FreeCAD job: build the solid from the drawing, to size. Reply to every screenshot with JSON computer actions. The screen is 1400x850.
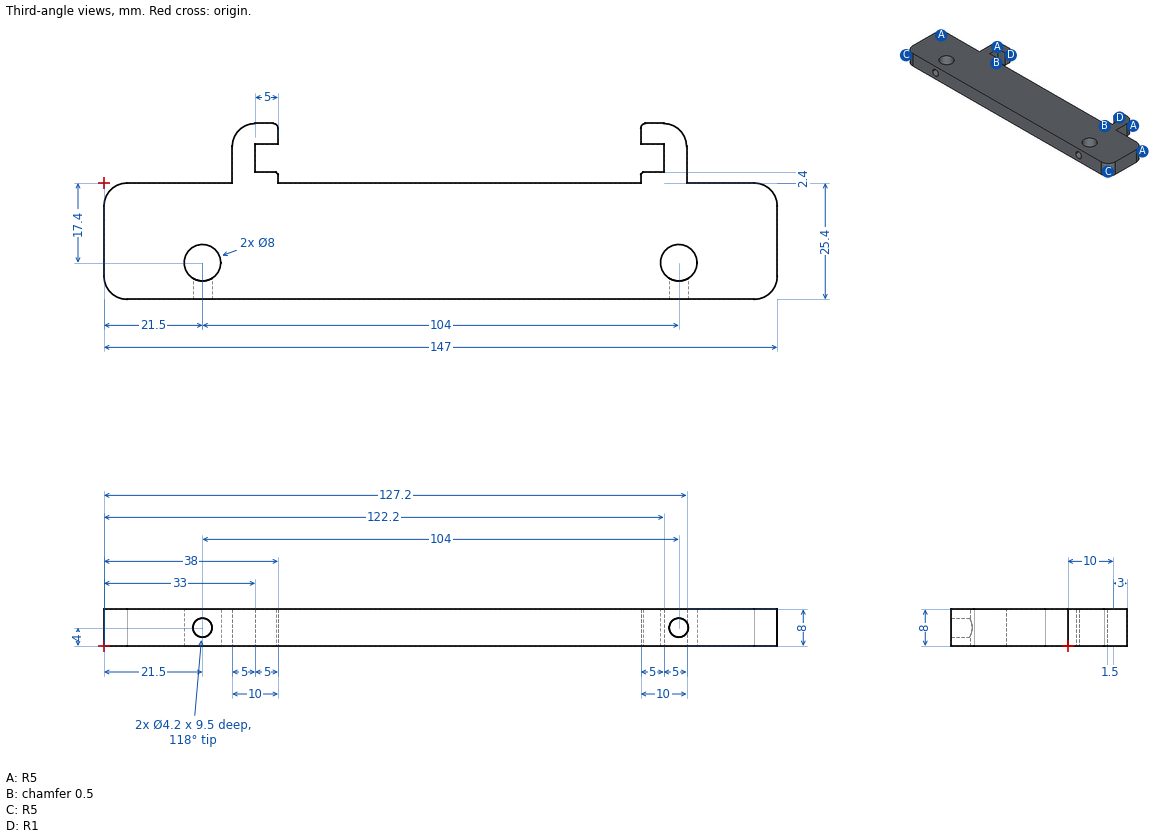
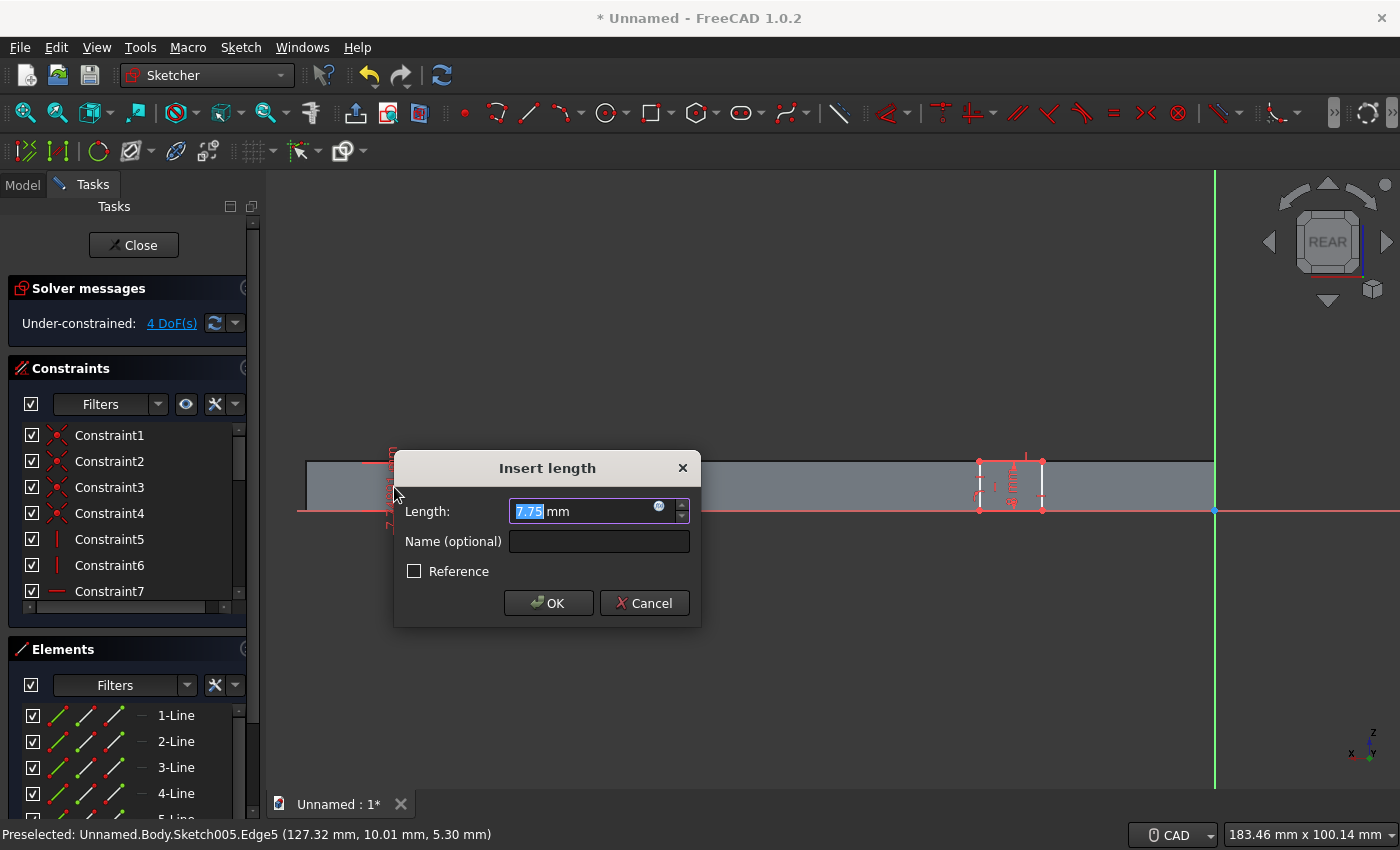
{"action": "type", "text": "8"}
{"action": "key", "text": "Return"}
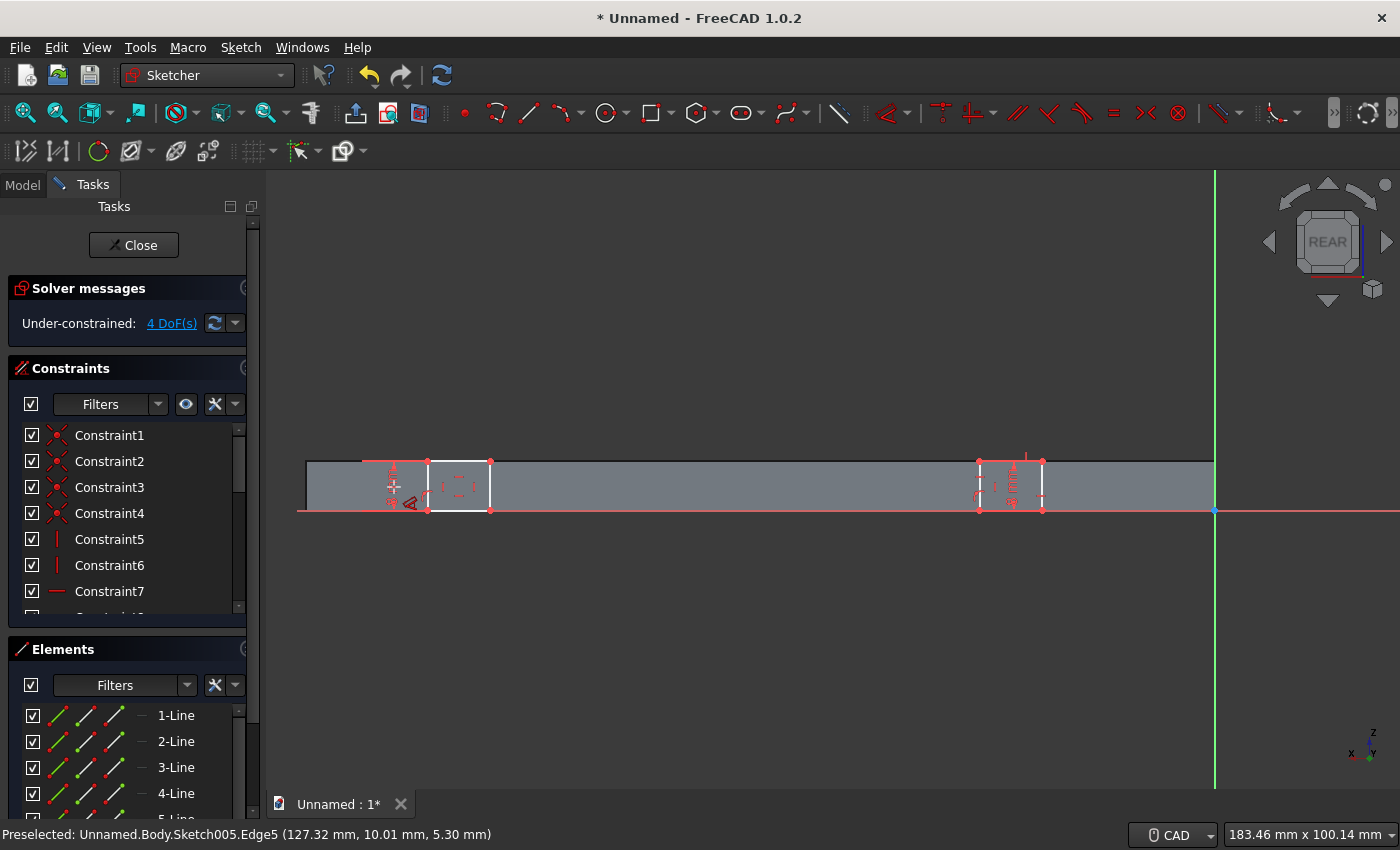
{"action": "left_click", "coordinate": [998, 511]}
{"action": "left_click", "coordinate": [1011, 545]}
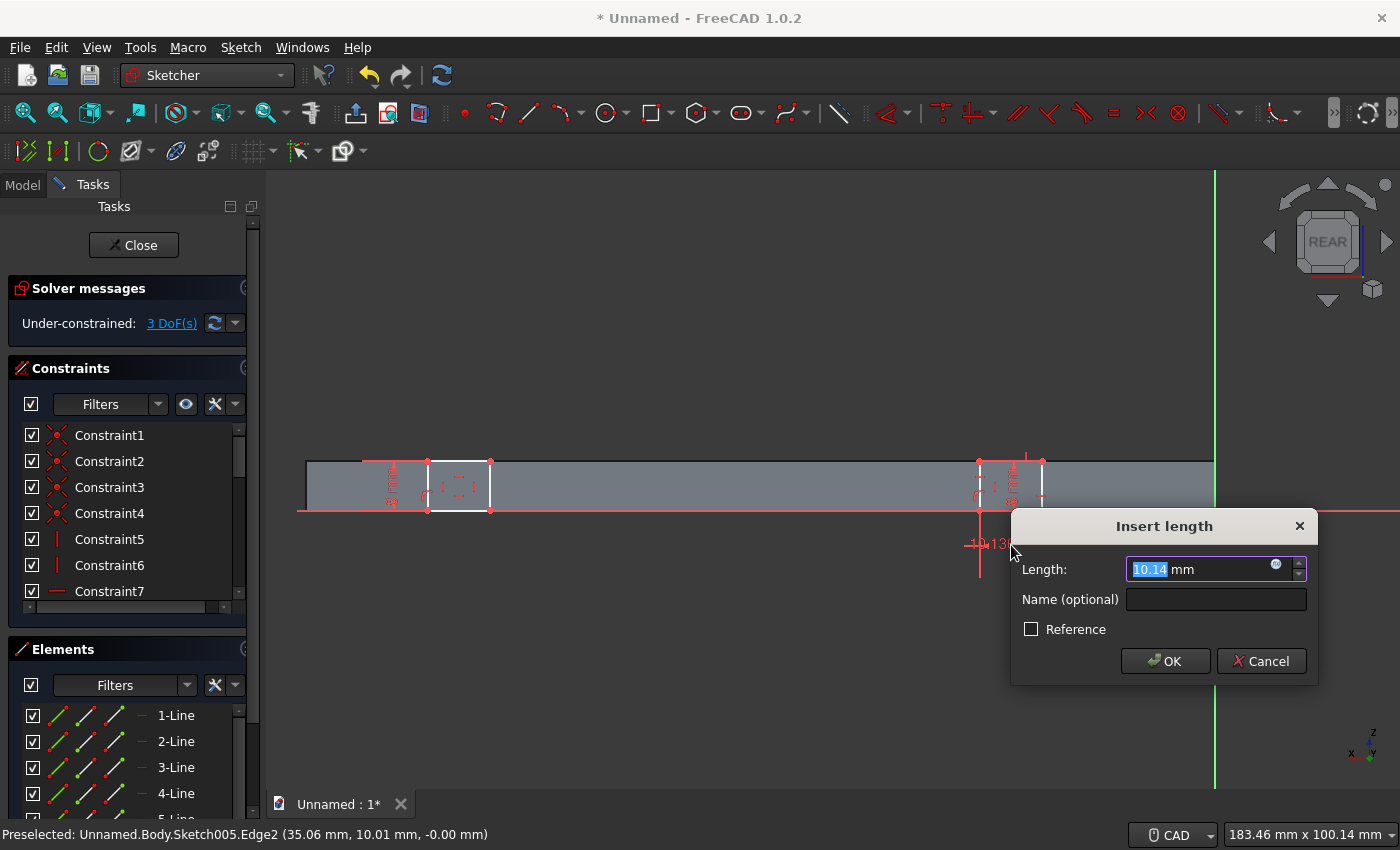
{"action": "type", "text": "10"}
{"action": "key", "text": "Return"}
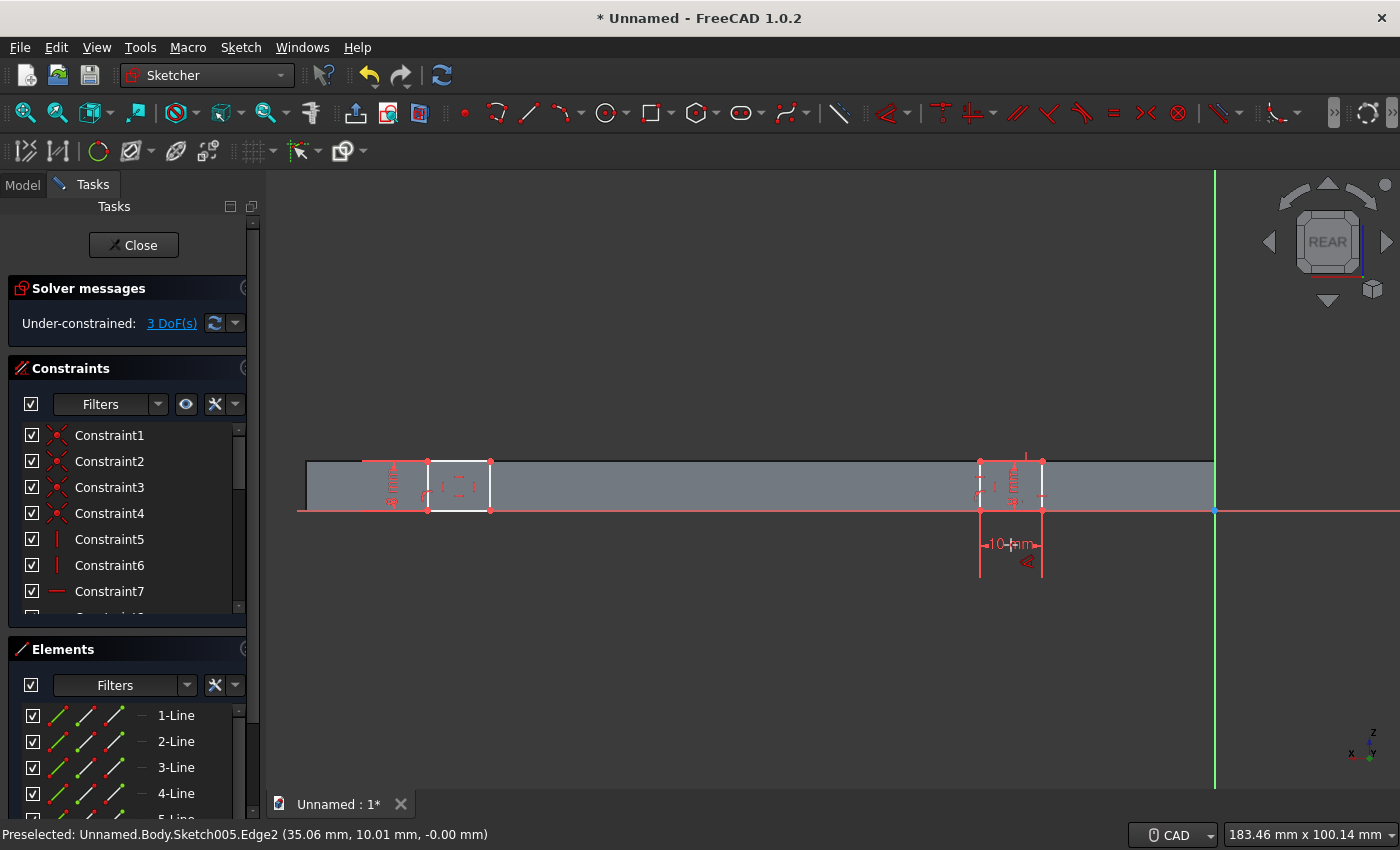
{"action": "left_click", "coordinate": [447, 511]}
{"action": "left_click", "coordinate": [459, 545]}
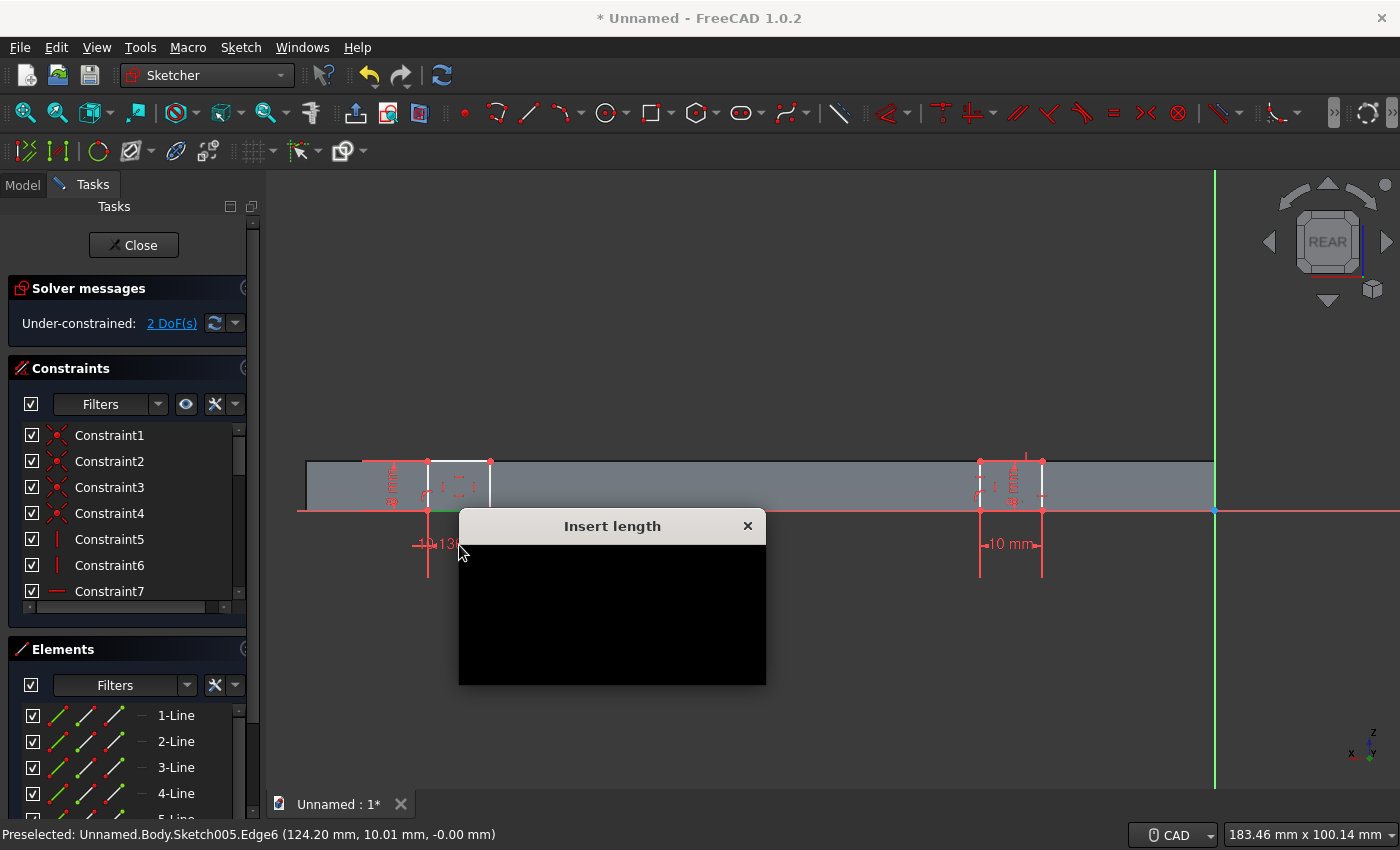
{"action": "type", "text": "10"}
{"action": "key", "text": "Return"}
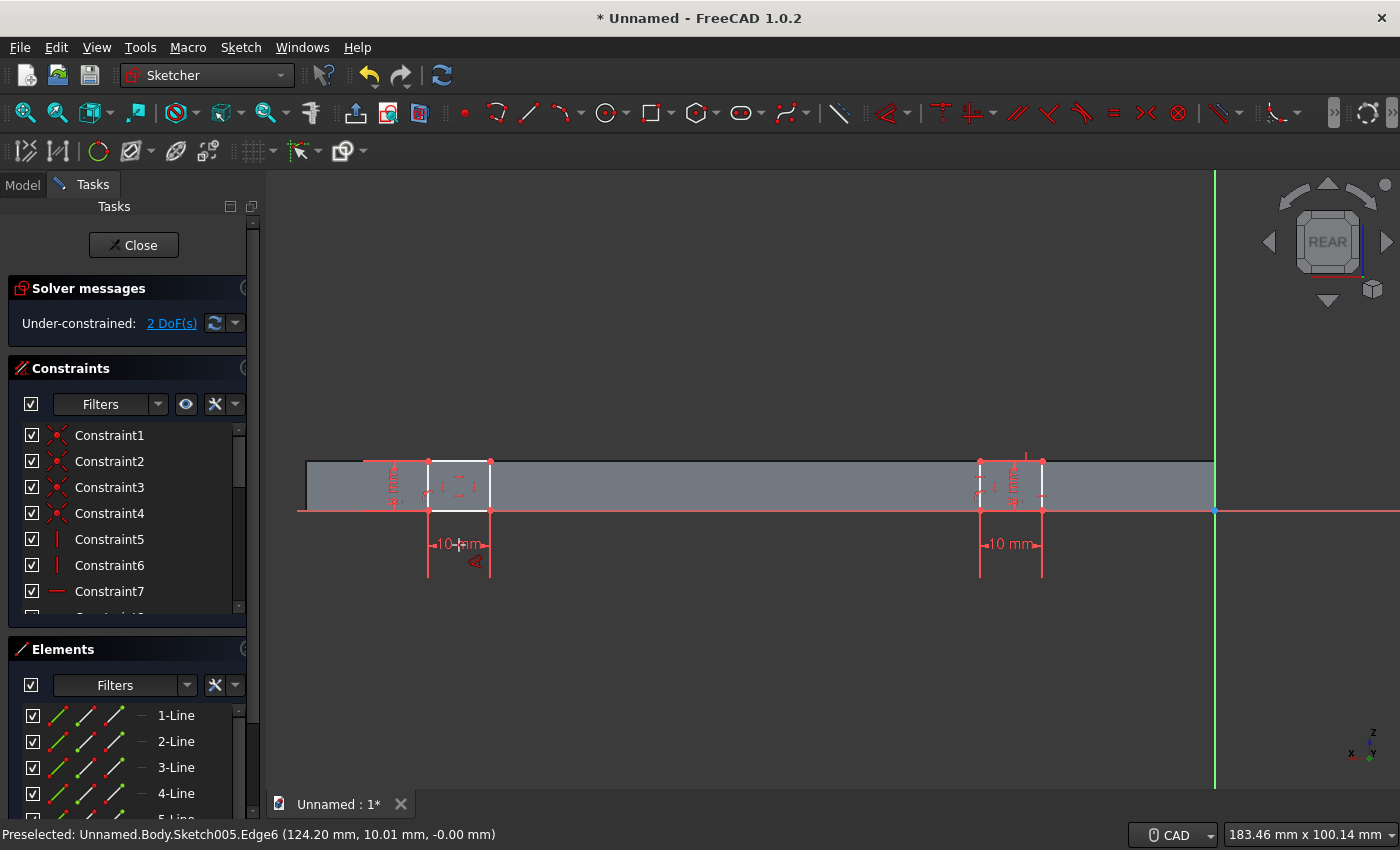
{"action": "left_click", "coordinate": [980, 461]}
{"action": "left_click", "coordinate": [1097, 545]}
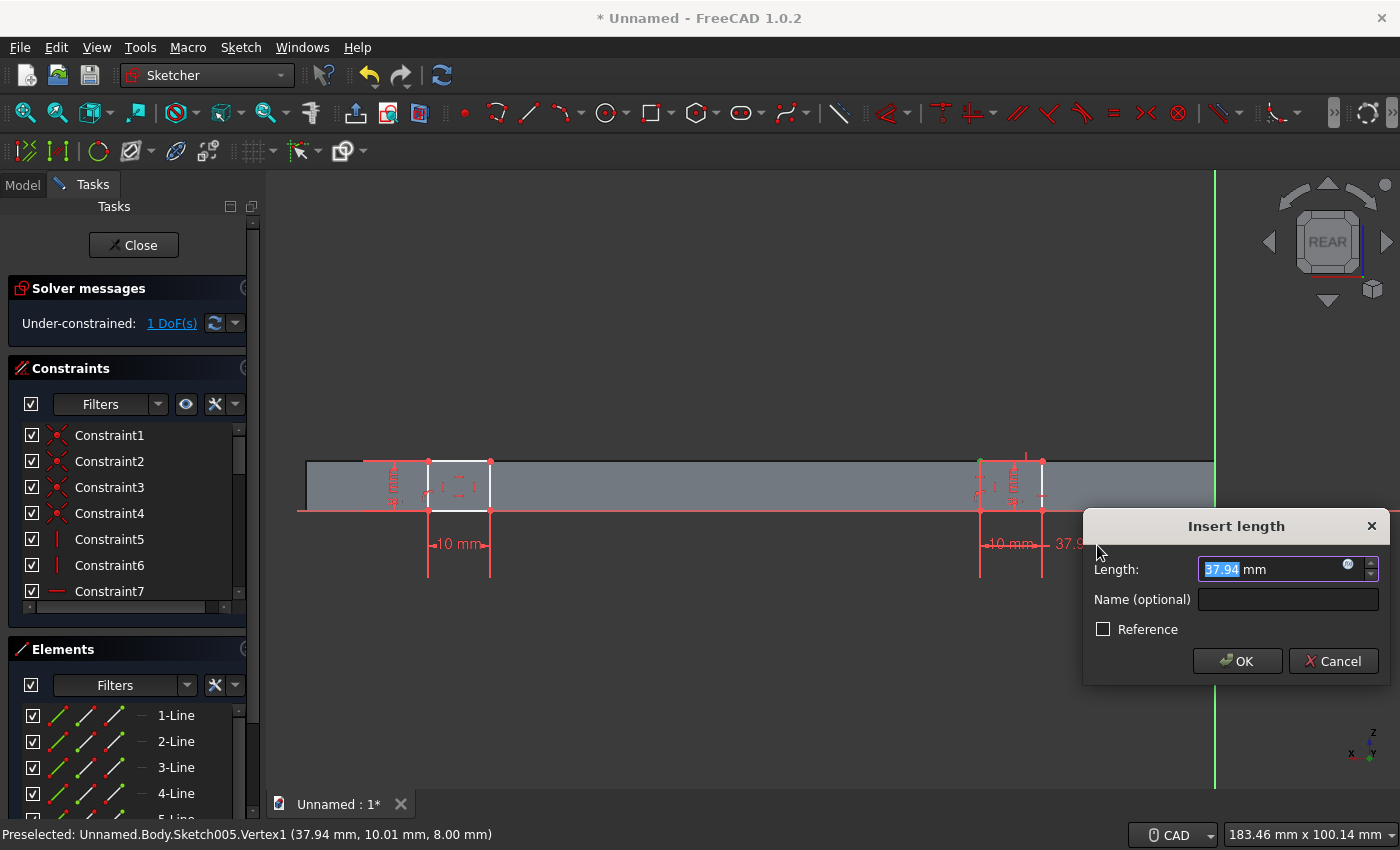
{"action": "type", "text": "38"}
{"action": "key", "text": "Return"}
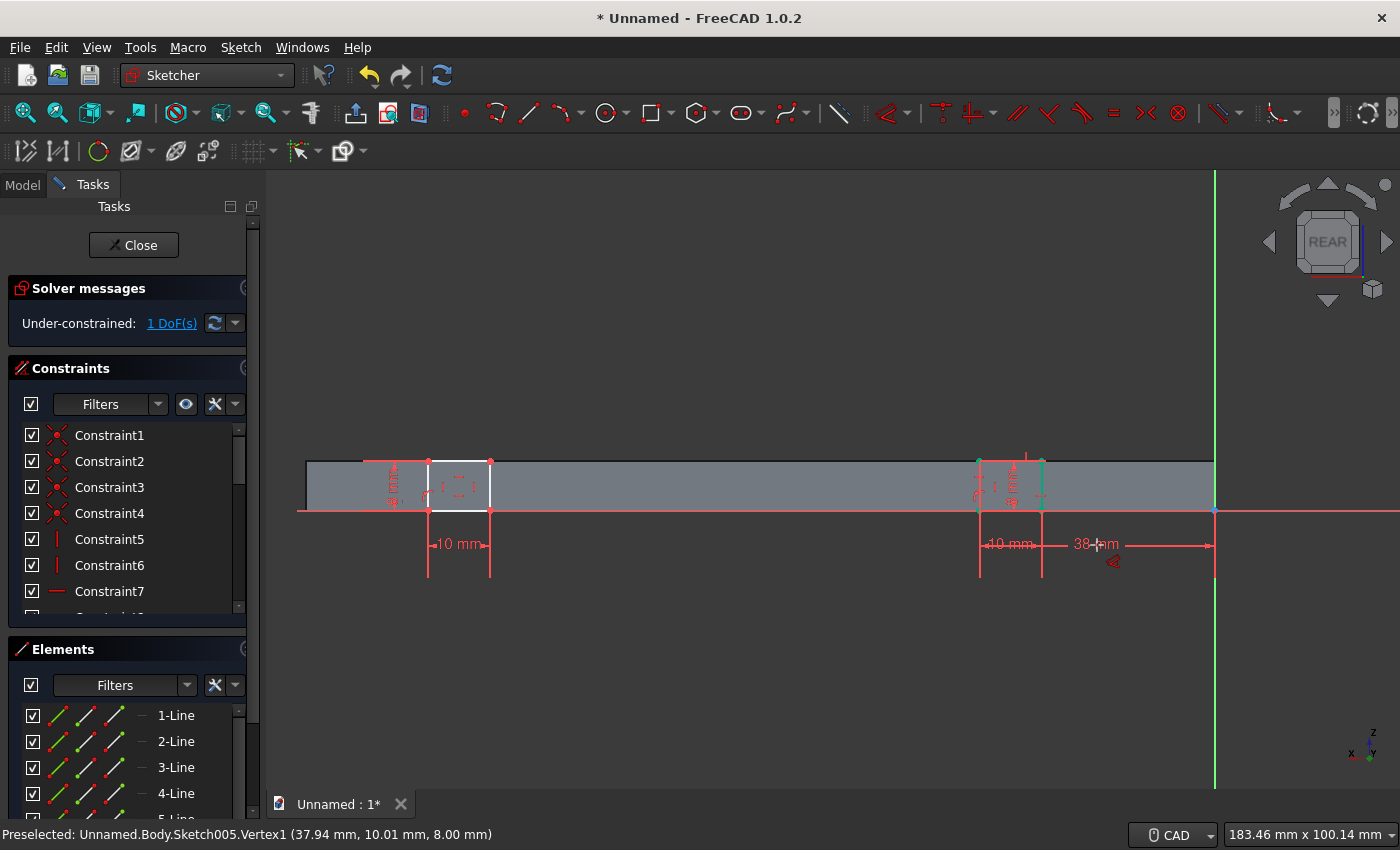
{"action": "left_click", "coordinate": [428, 461]}
{"action": "left_click", "coordinate": [821, 545]}